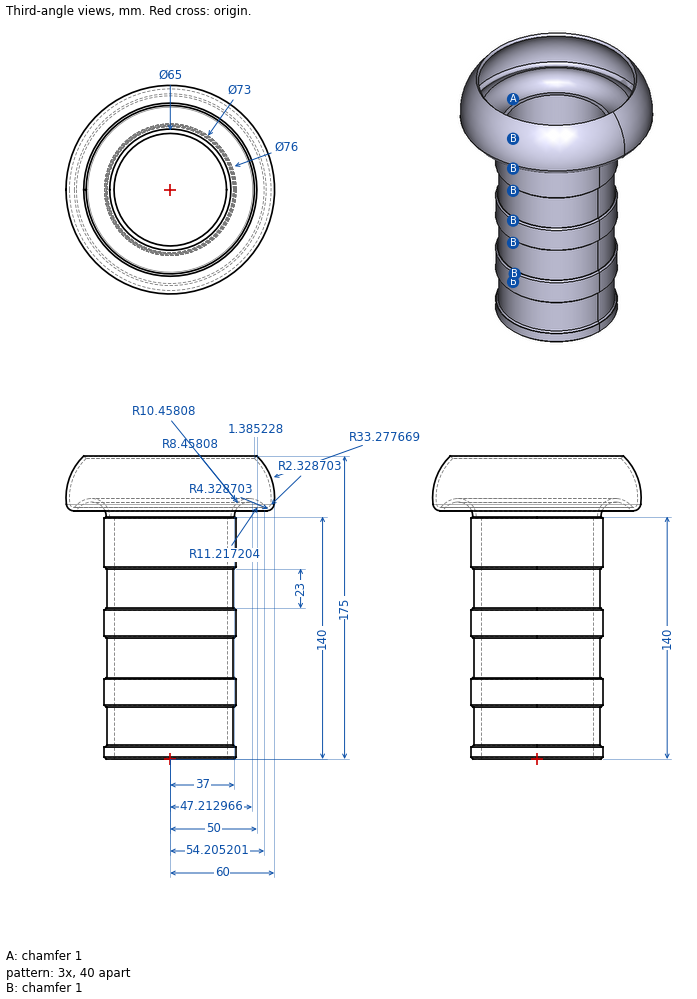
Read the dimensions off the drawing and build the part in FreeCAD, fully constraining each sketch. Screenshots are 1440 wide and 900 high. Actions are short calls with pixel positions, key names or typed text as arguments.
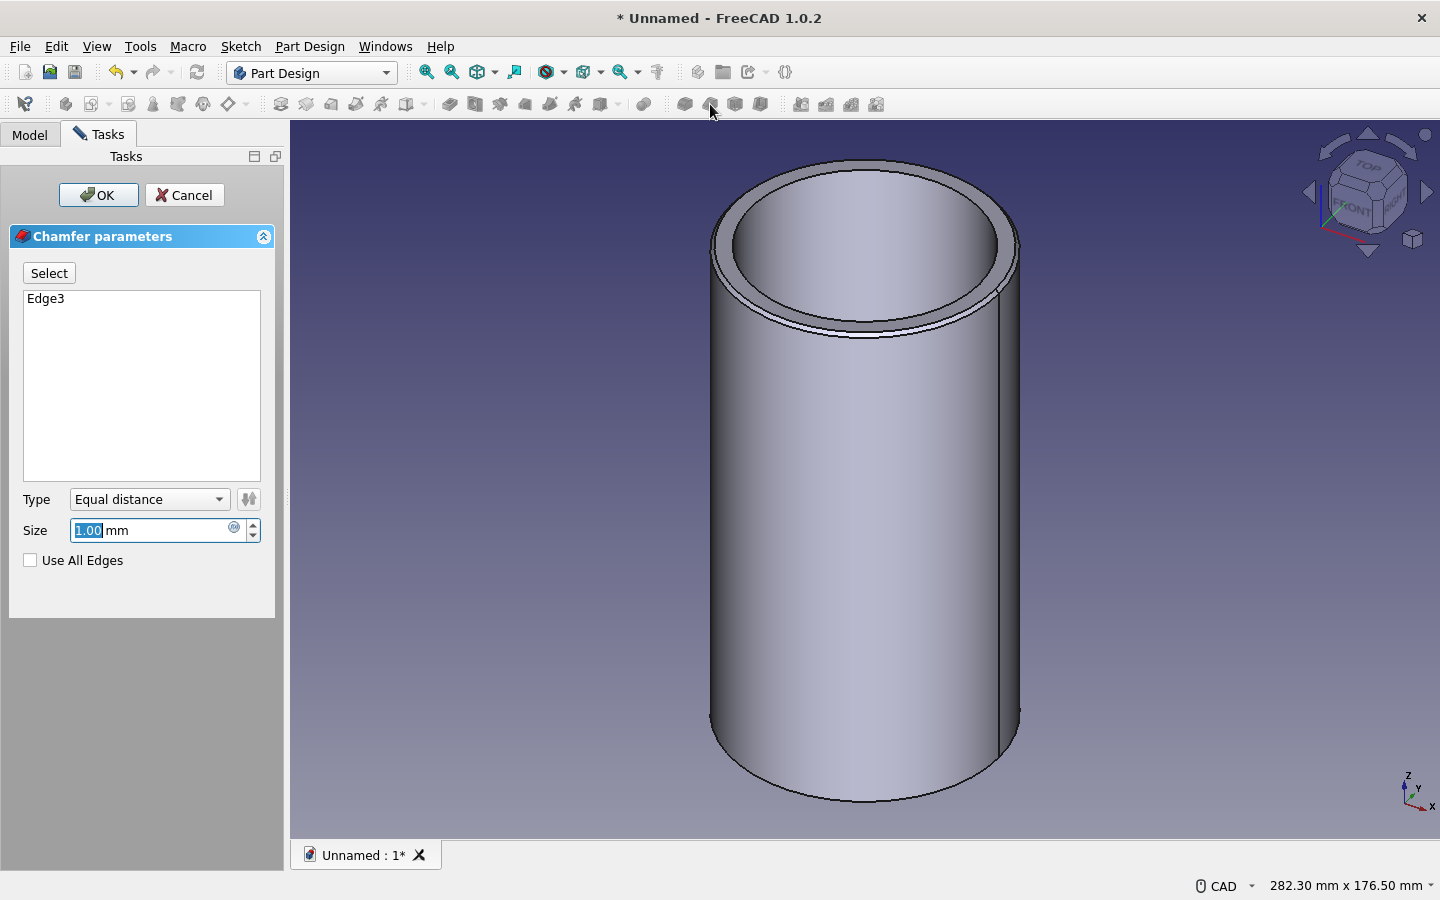
text(1)
key(Tab)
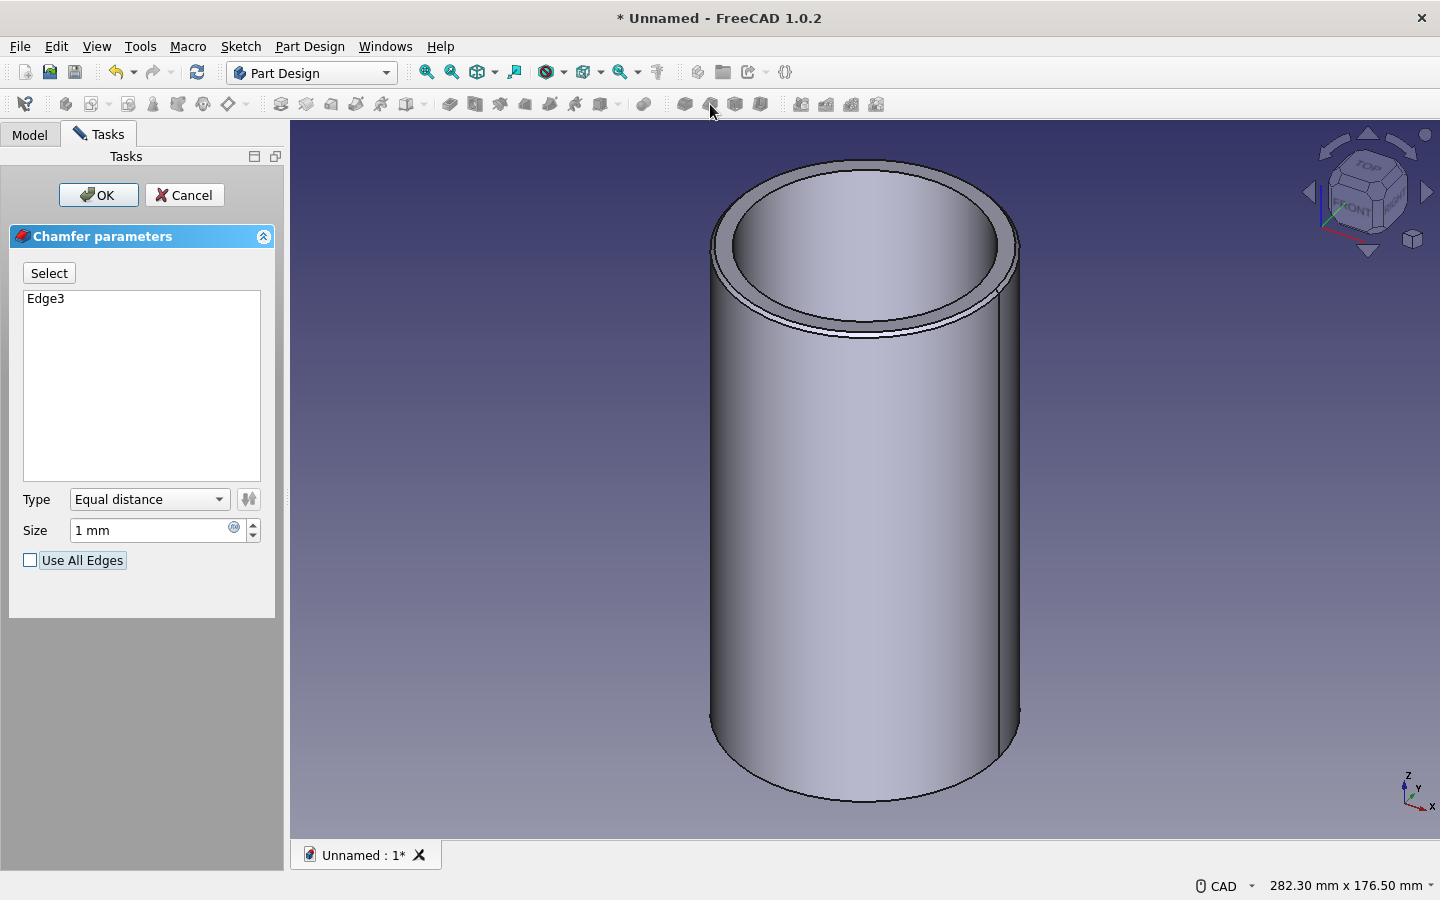
click(99, 195)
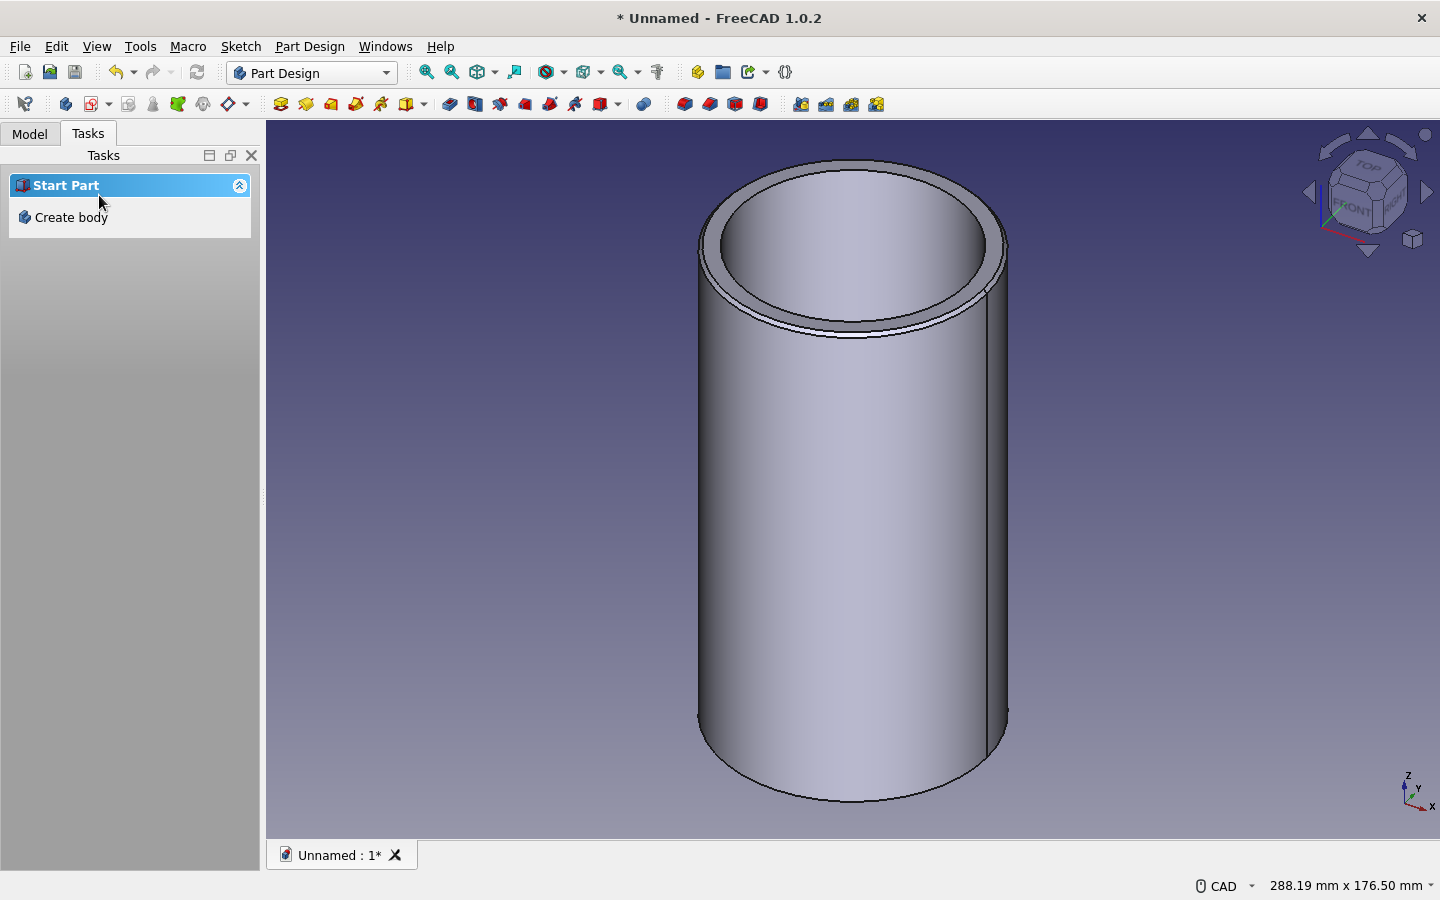
click(30, 134)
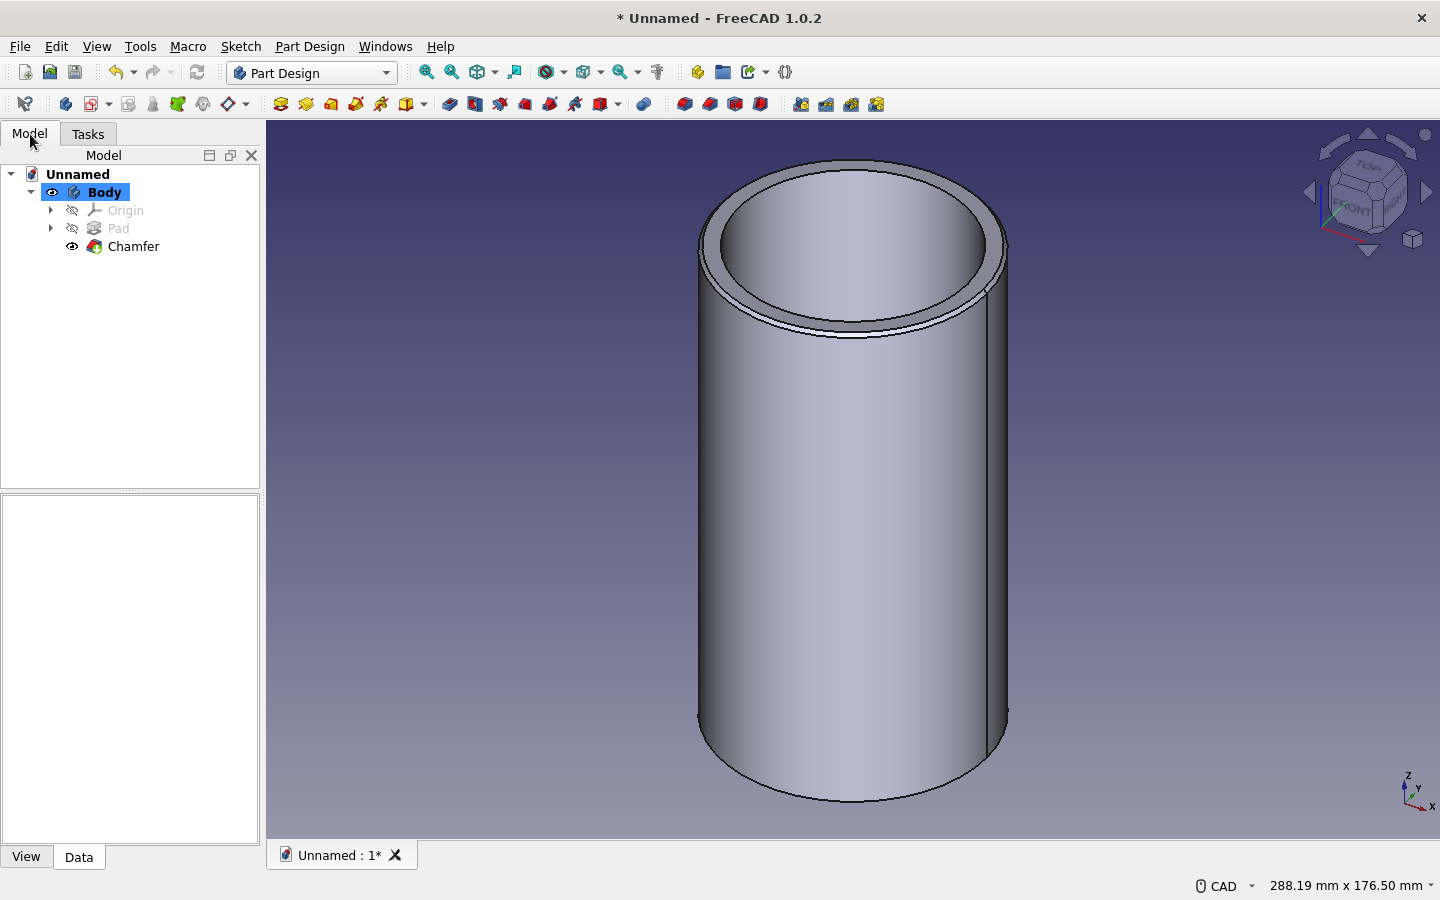
click(51, 210)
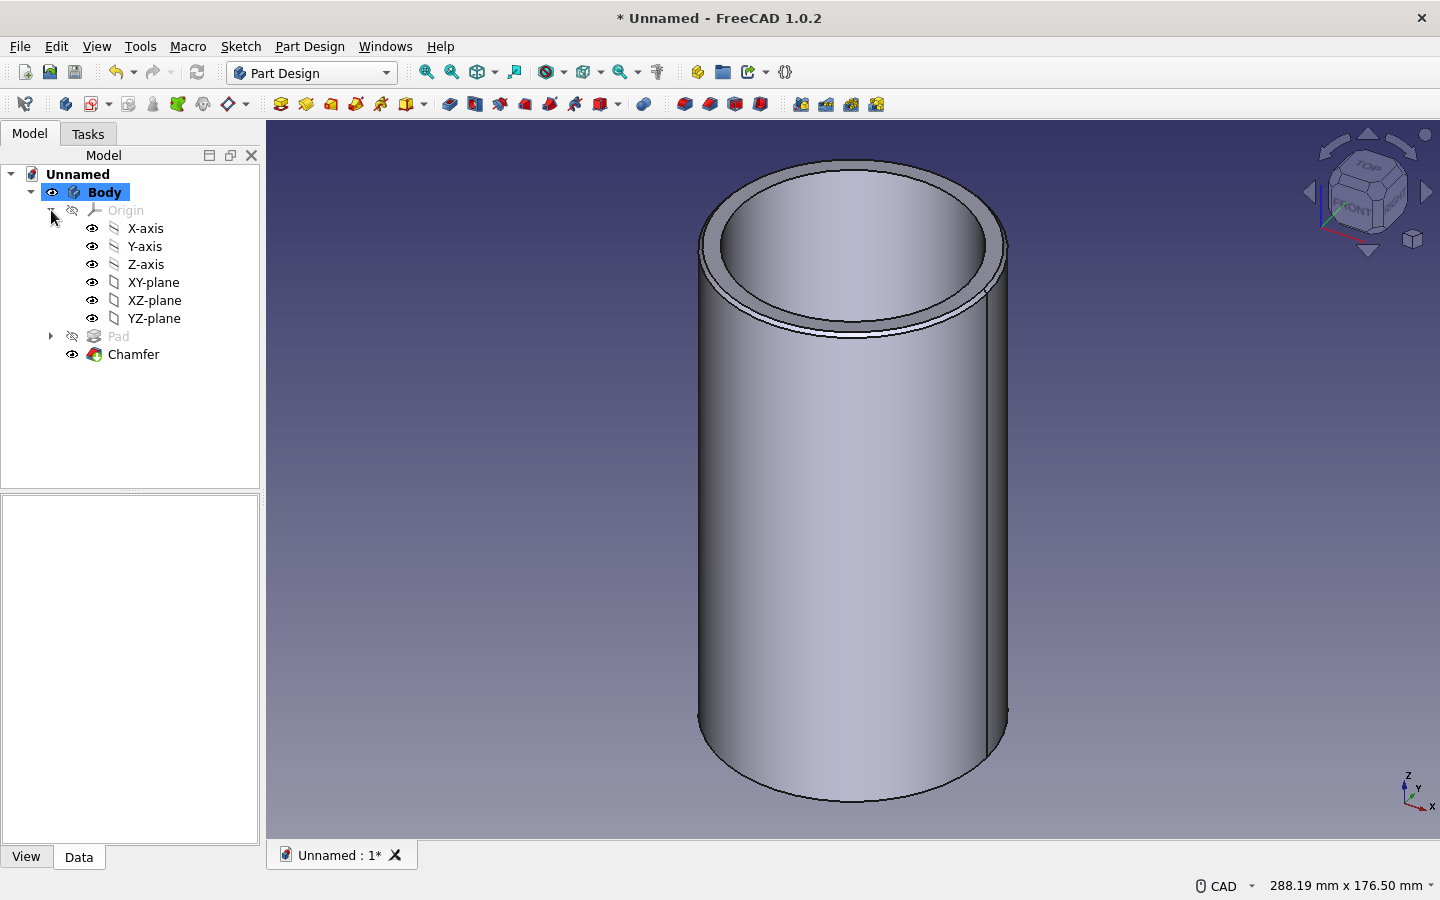
click(137, 282)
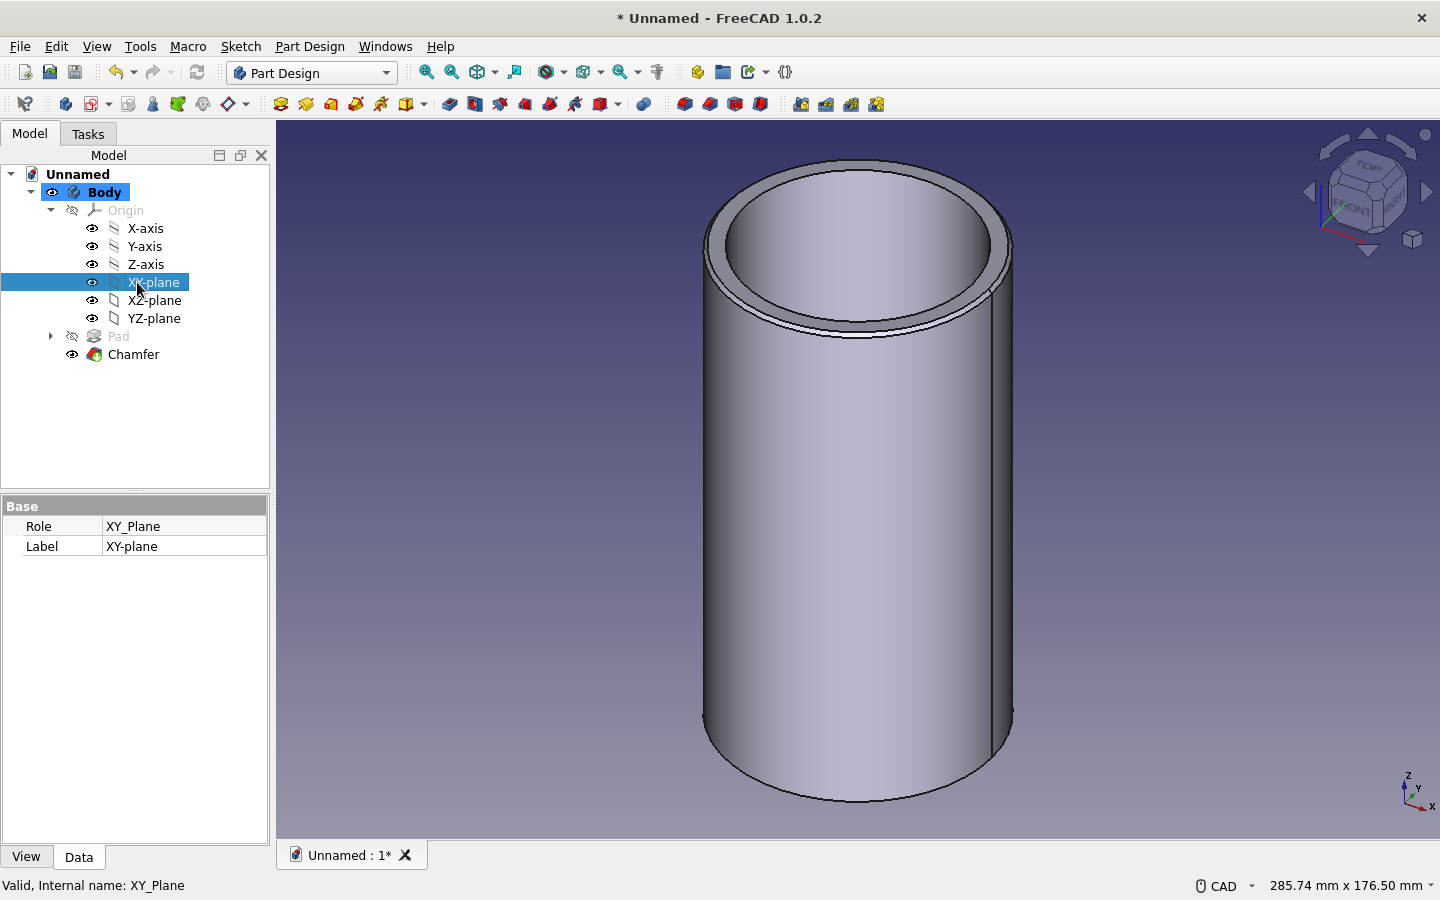
click(228, 104)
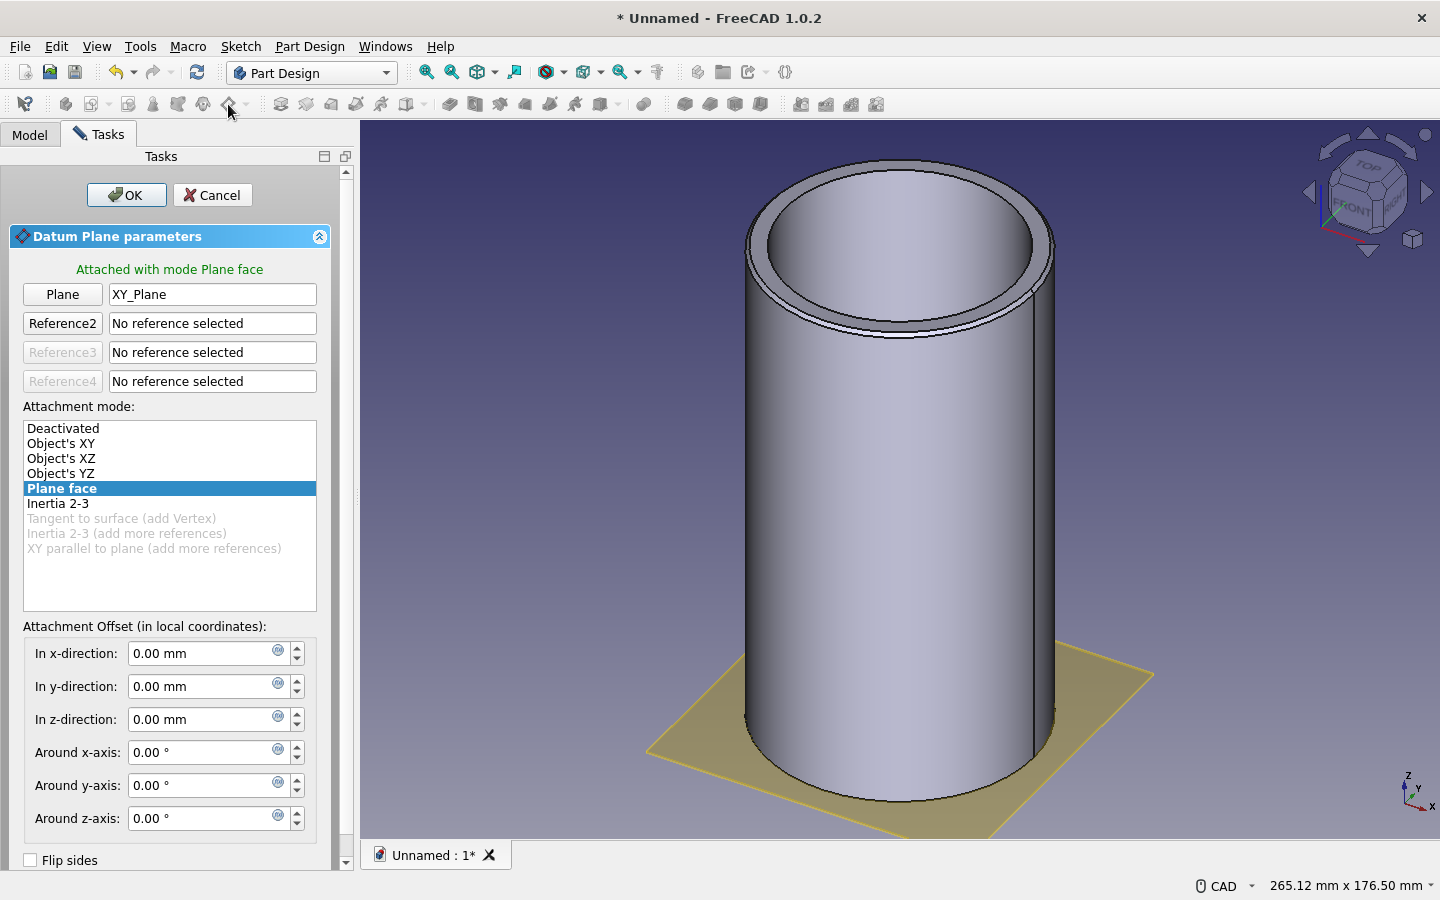
triple_click(210, 720)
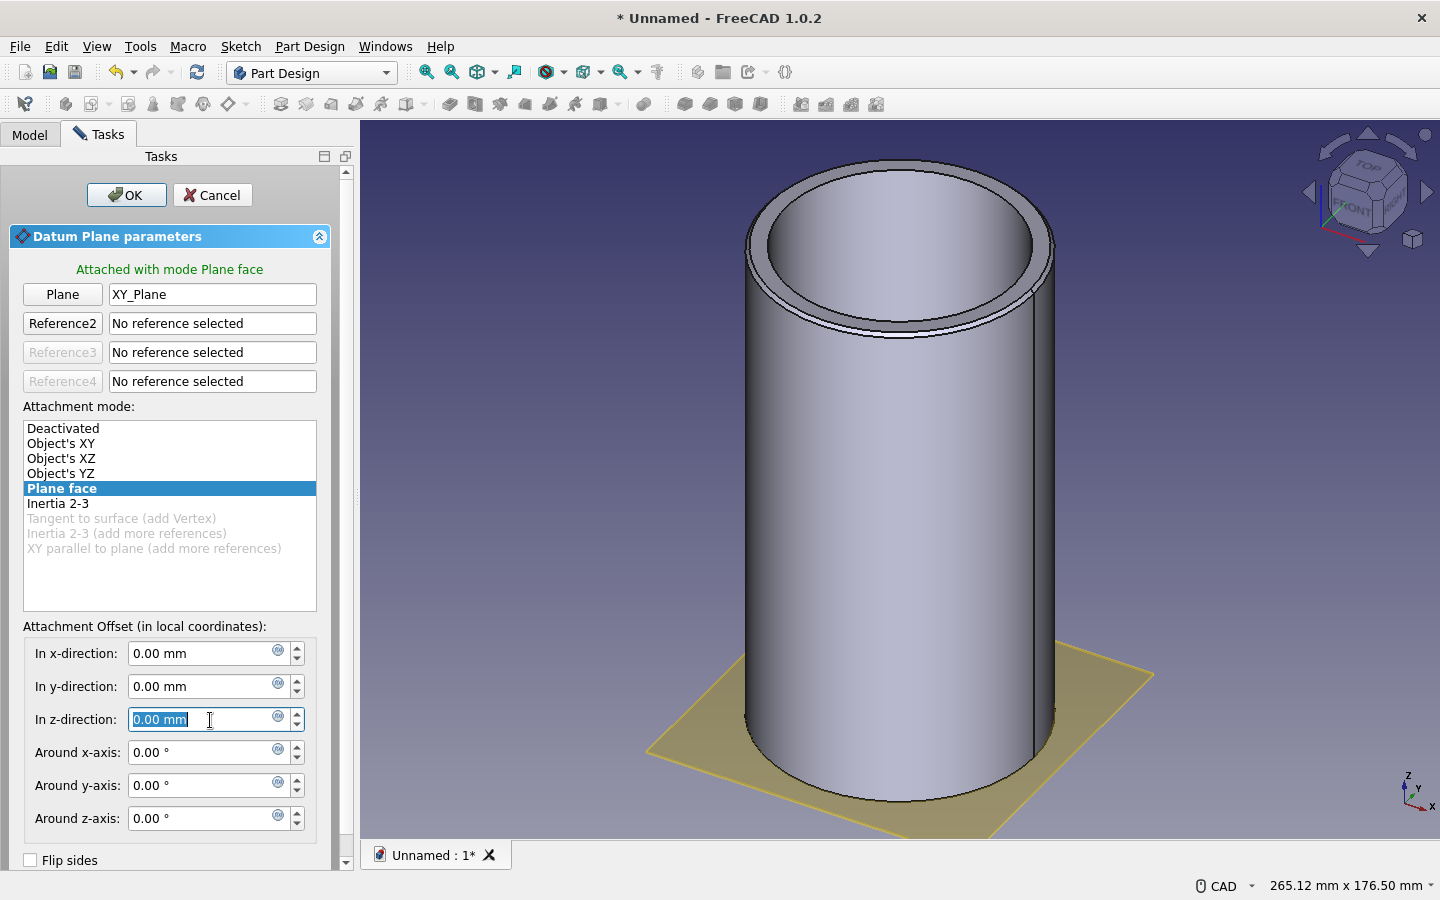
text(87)
key(Tab)